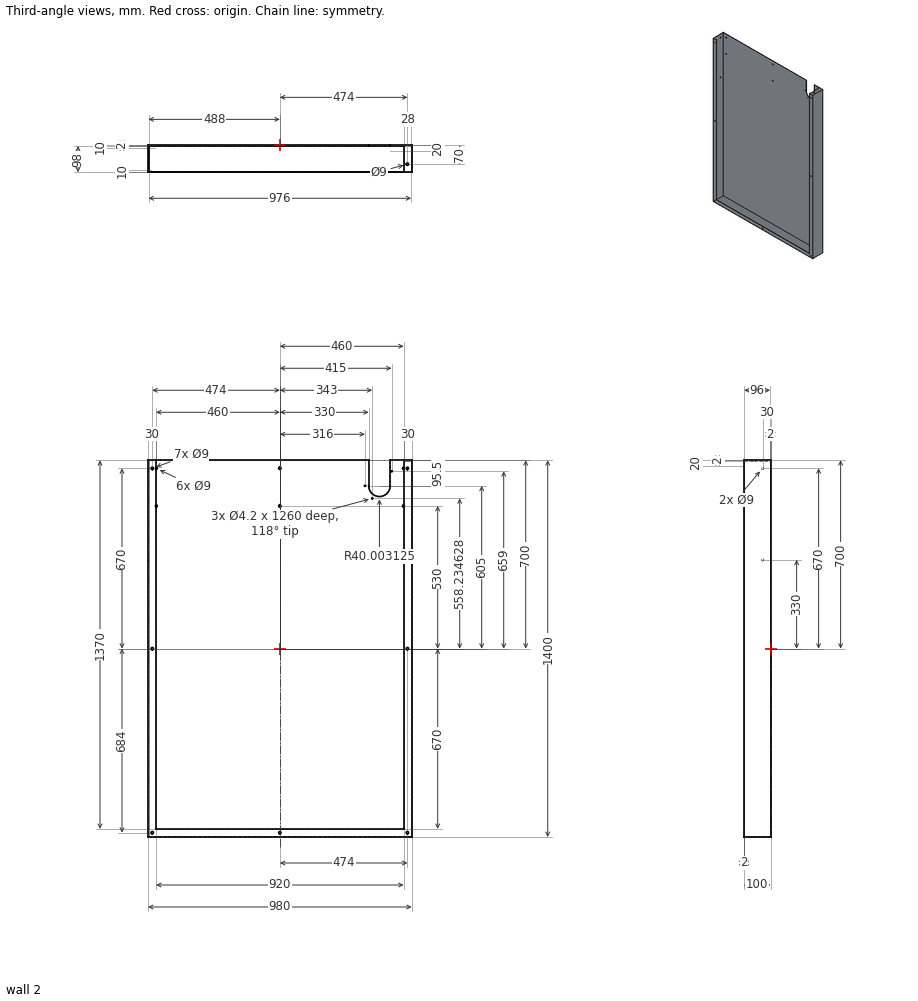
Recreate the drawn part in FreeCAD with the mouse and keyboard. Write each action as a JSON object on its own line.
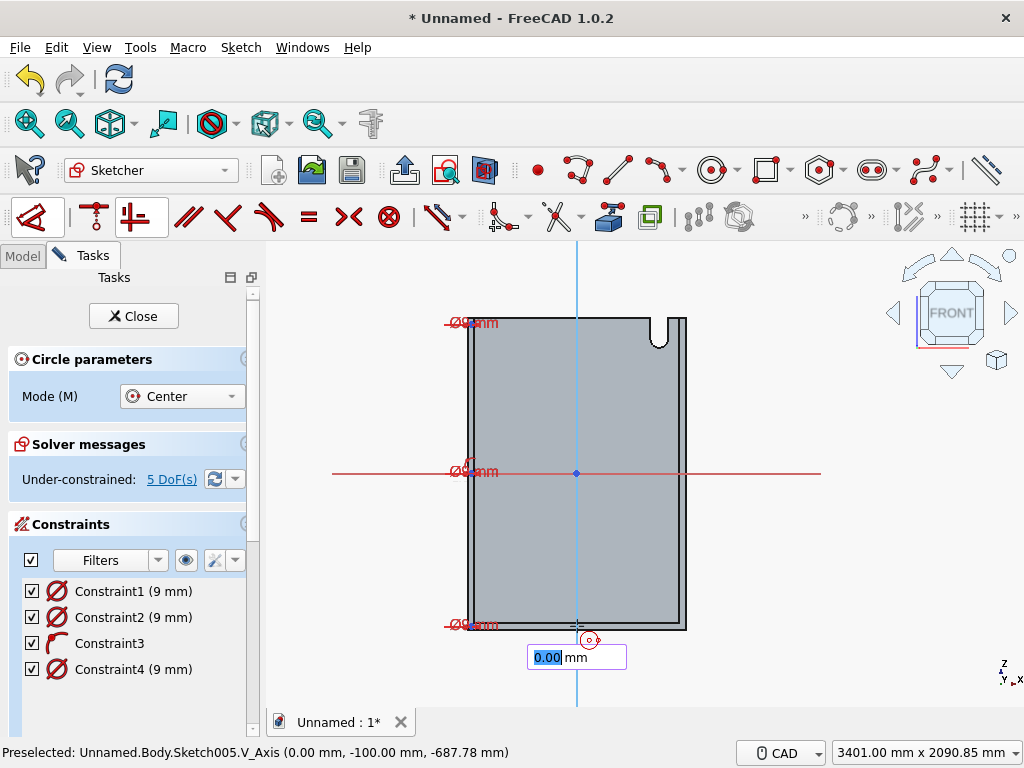
{"action": "scroll", "coordinate": [578, 626], "scroll_direction": "up", "scroll_amount": 15}
{"action": "mouse_move", "coordinate": [565, 606]}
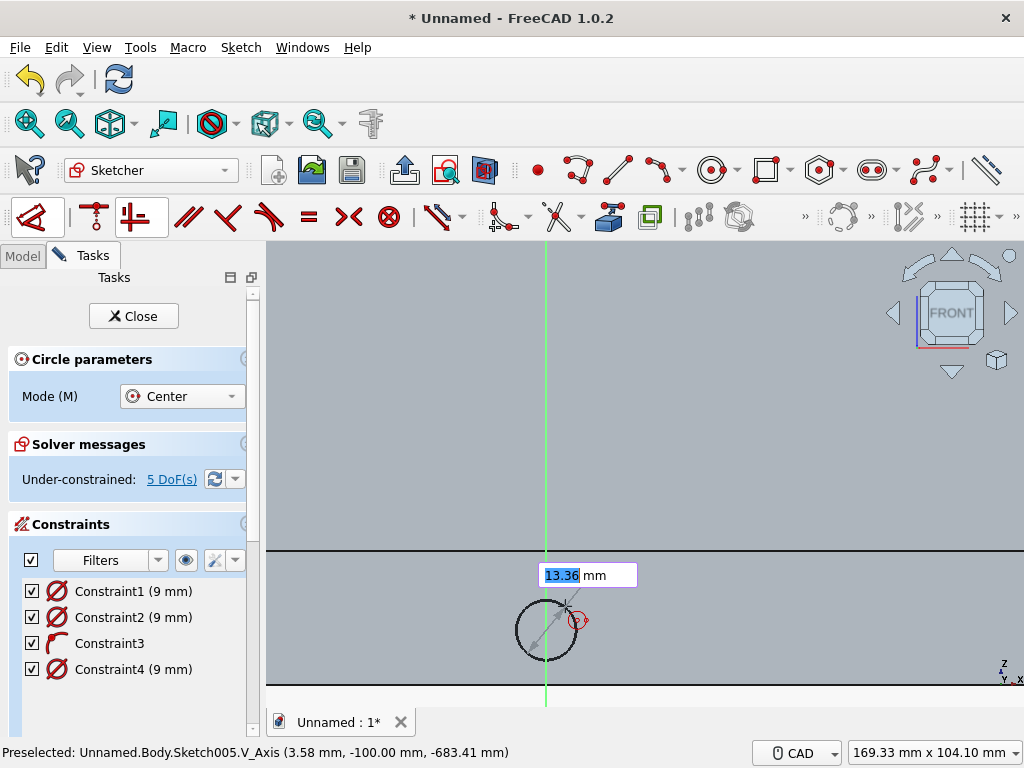
{"action": "type", "text": "9"}
{"action": "key", "text": "Return"}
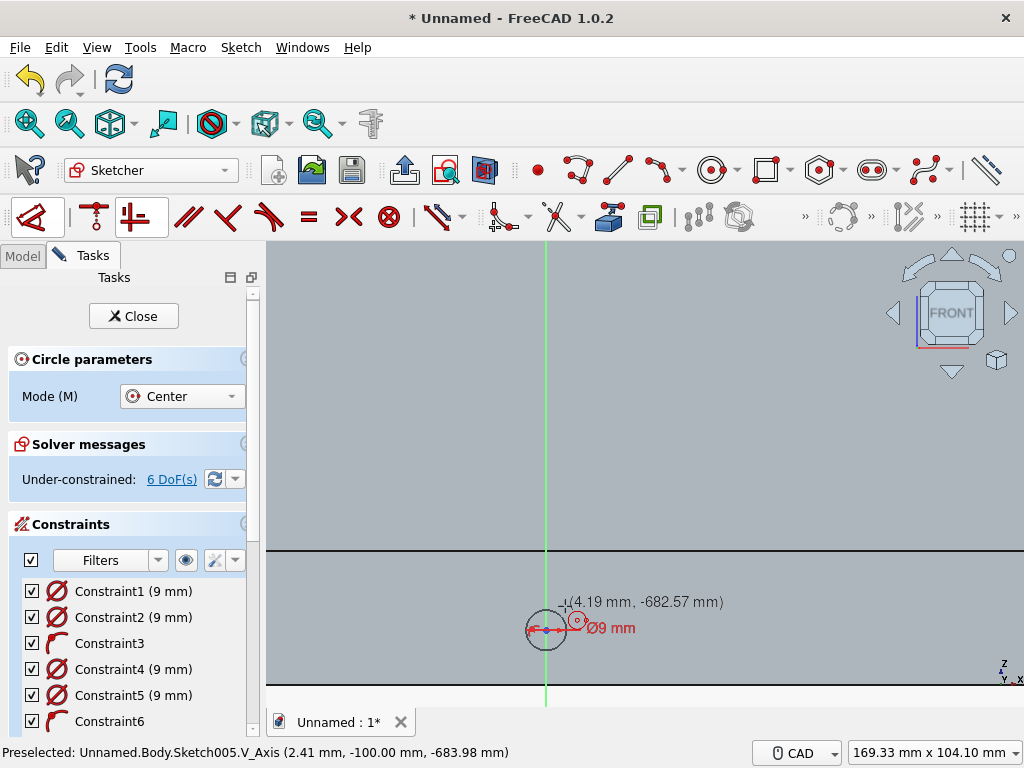
{"action": "scroll", "coordinate": [578, 625], "scroll_direction": "down", "scroll_amount": 15}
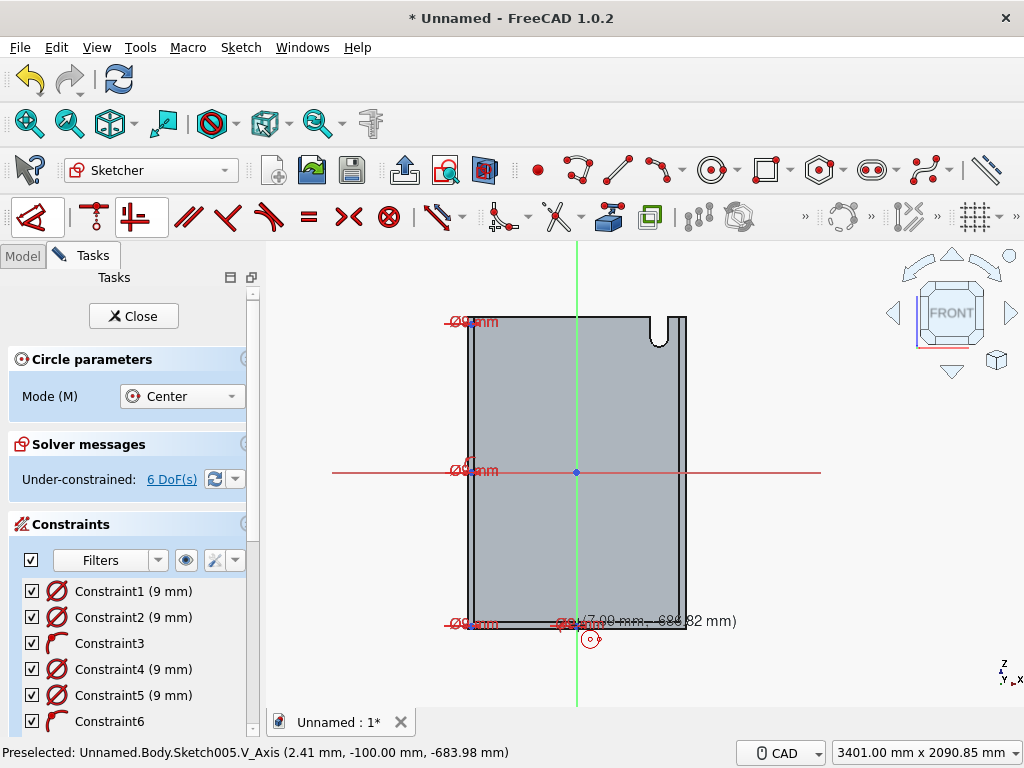
{"action": "scroll", "coordinate": [682, 625], "scroll_direction": "up", "scroll_amount": 16}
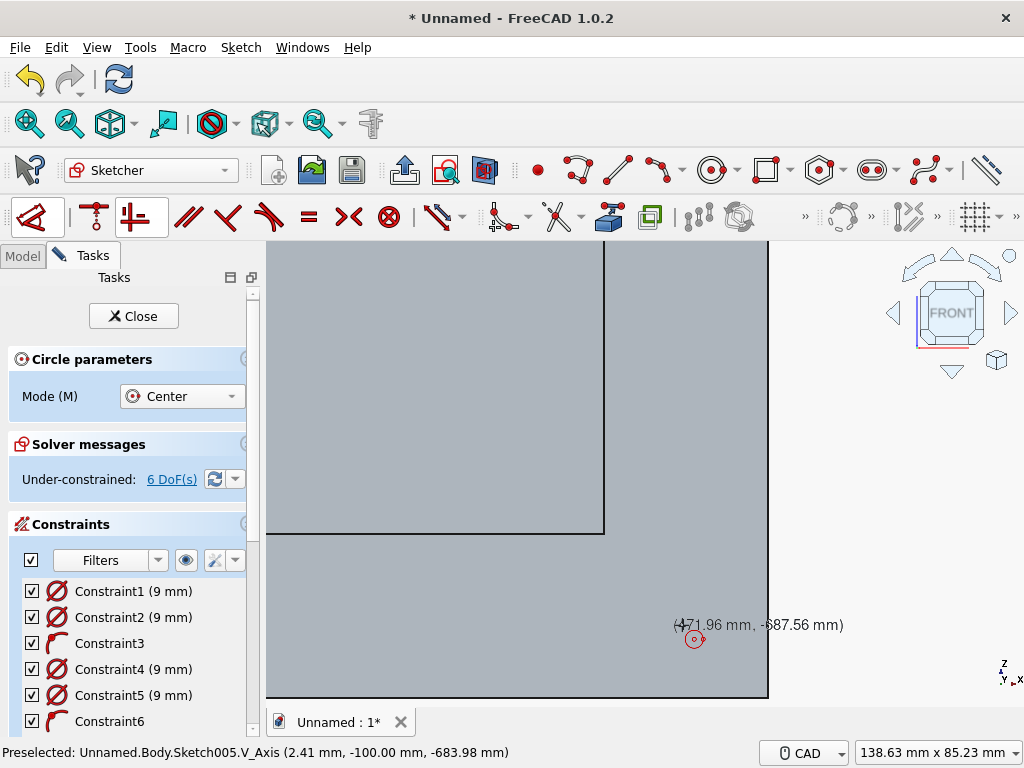
{"action": "scroll", "coordinate": [682, 625], "scroll_direction": "down", "scroll_amount": 16}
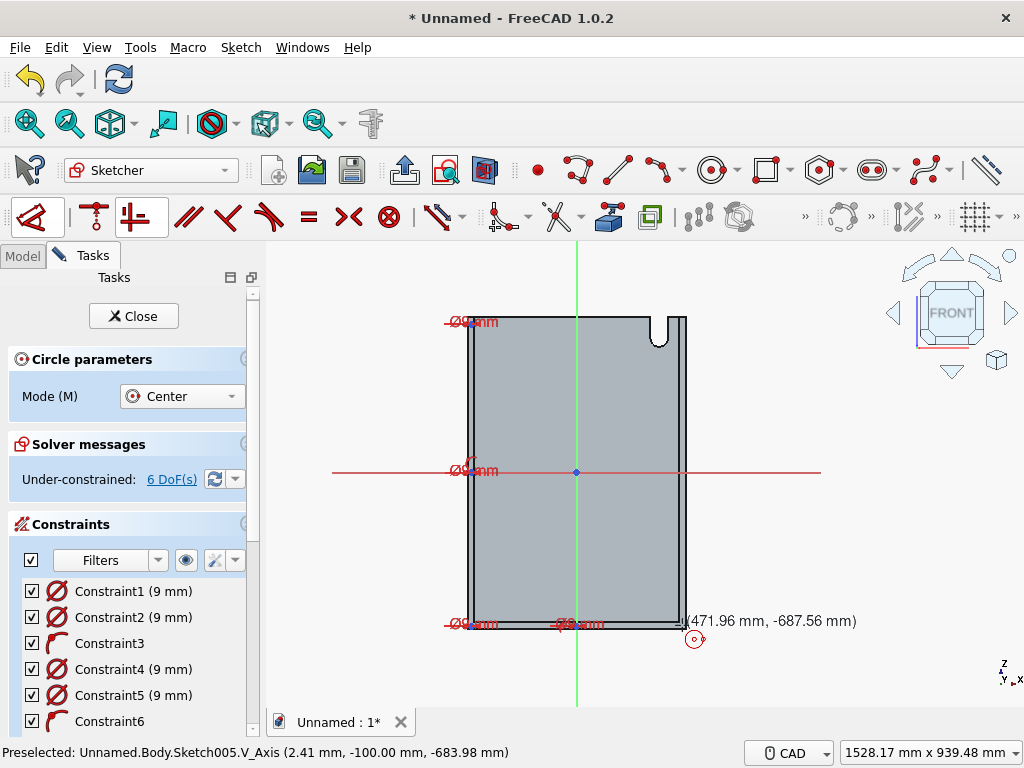
{"action": "left_click", "coordinate": [682, 625]}
{"action": "mouse_move", "coordinate": [683, 624]}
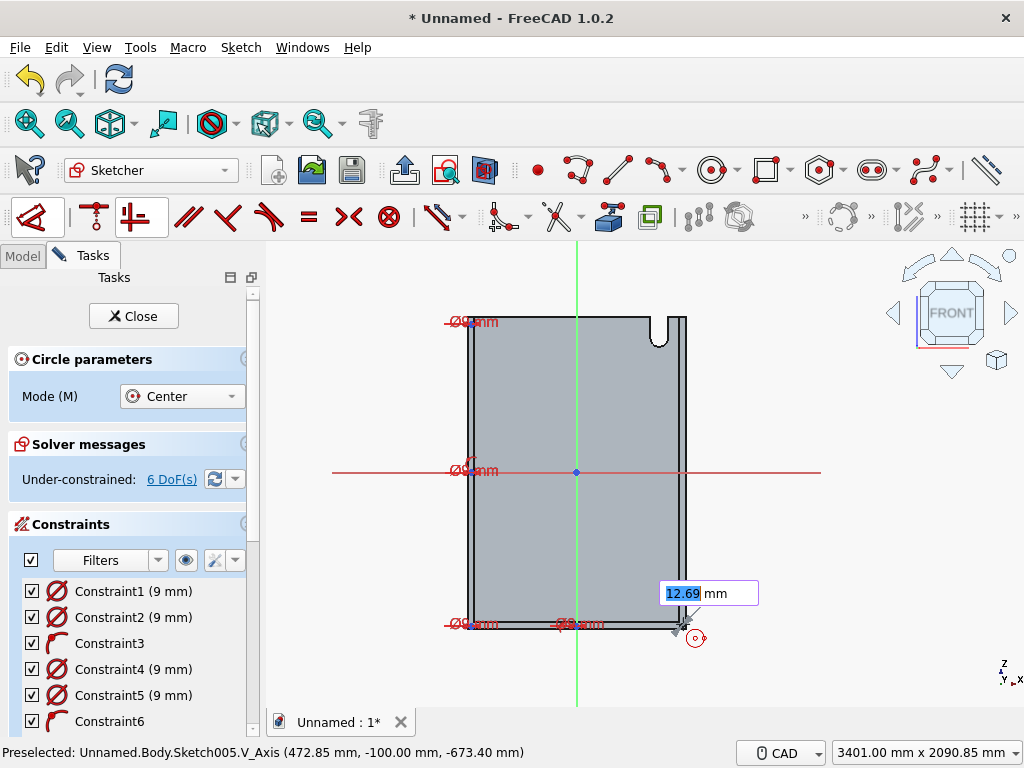
{"action": "type", "text": "9"}
{"action": "key", "text": "Return"}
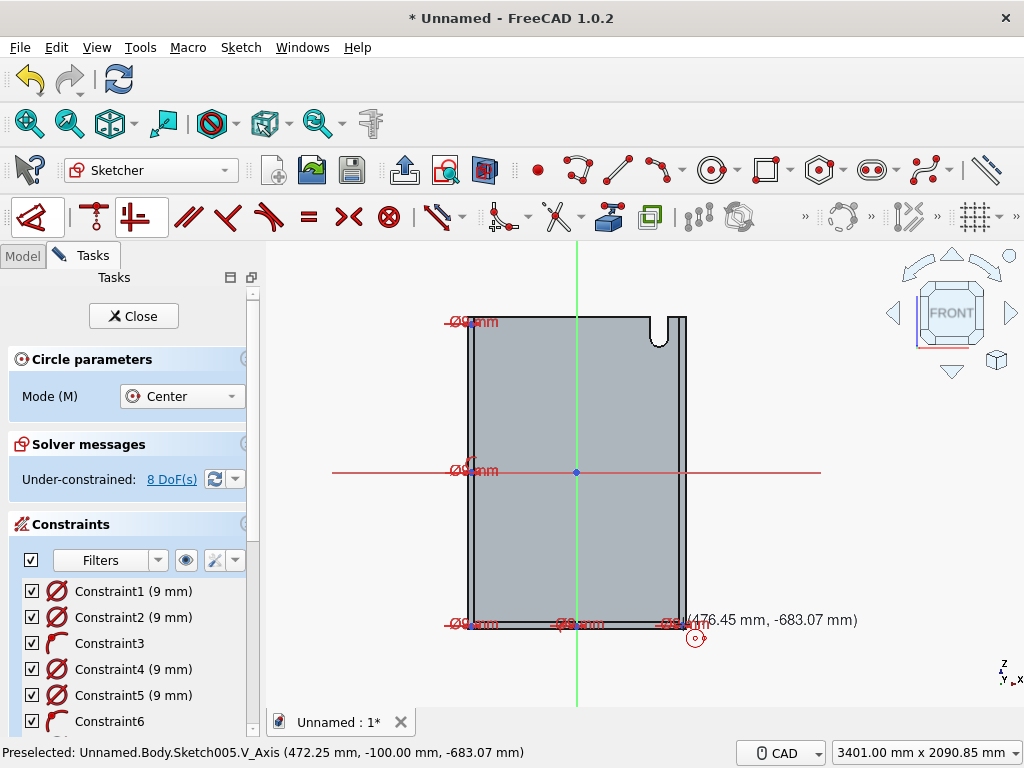
{"action": "scroll", "coordinate": [682, 473], "scroll_direction": "up", "scroll_amount": 16}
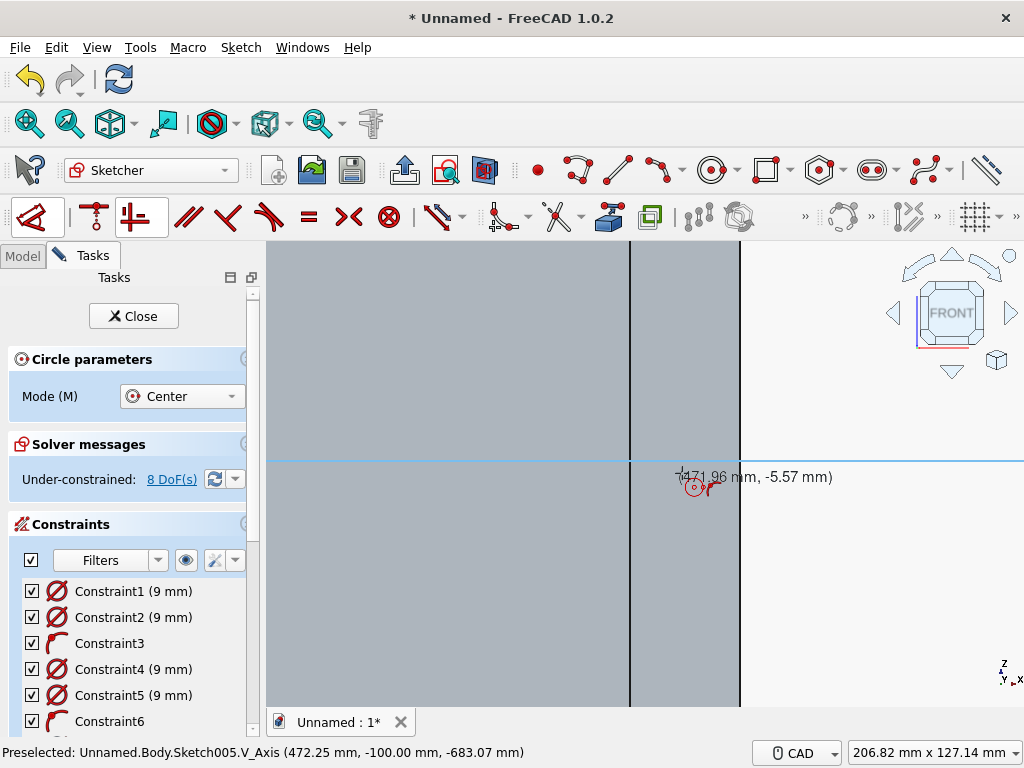
{"action": "scroll", "coordinate": [682, 473], "scroll_direction": "down", "scroll_amount": 16}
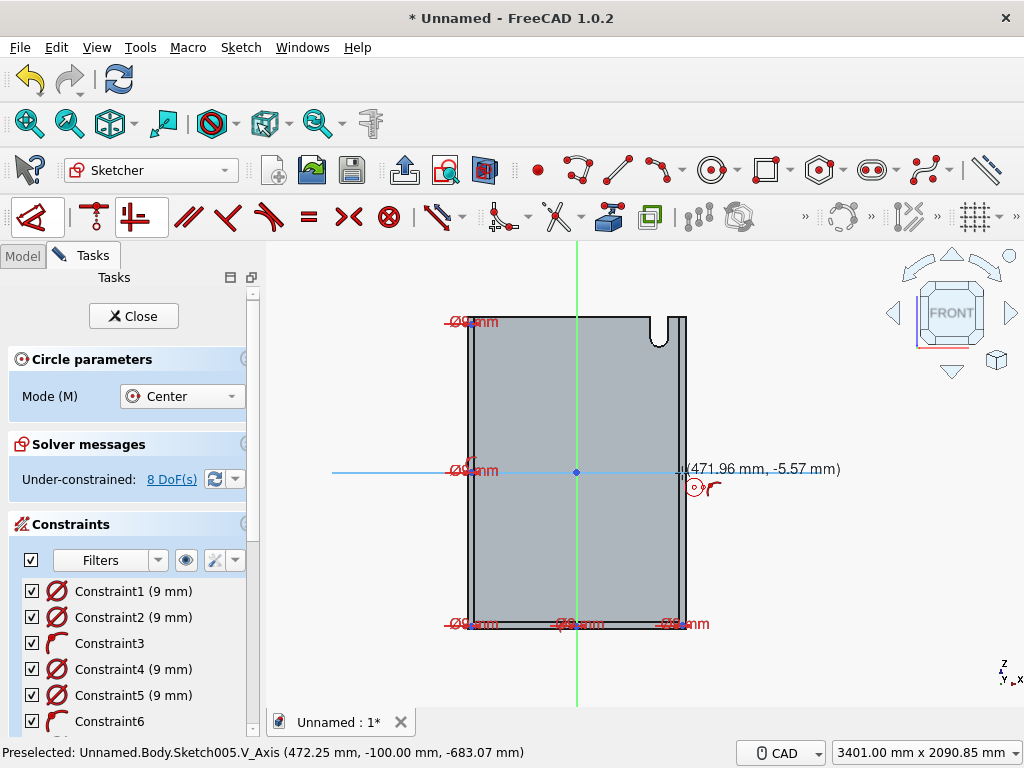
{"action": "left_click", "coordinate": [682, 473]}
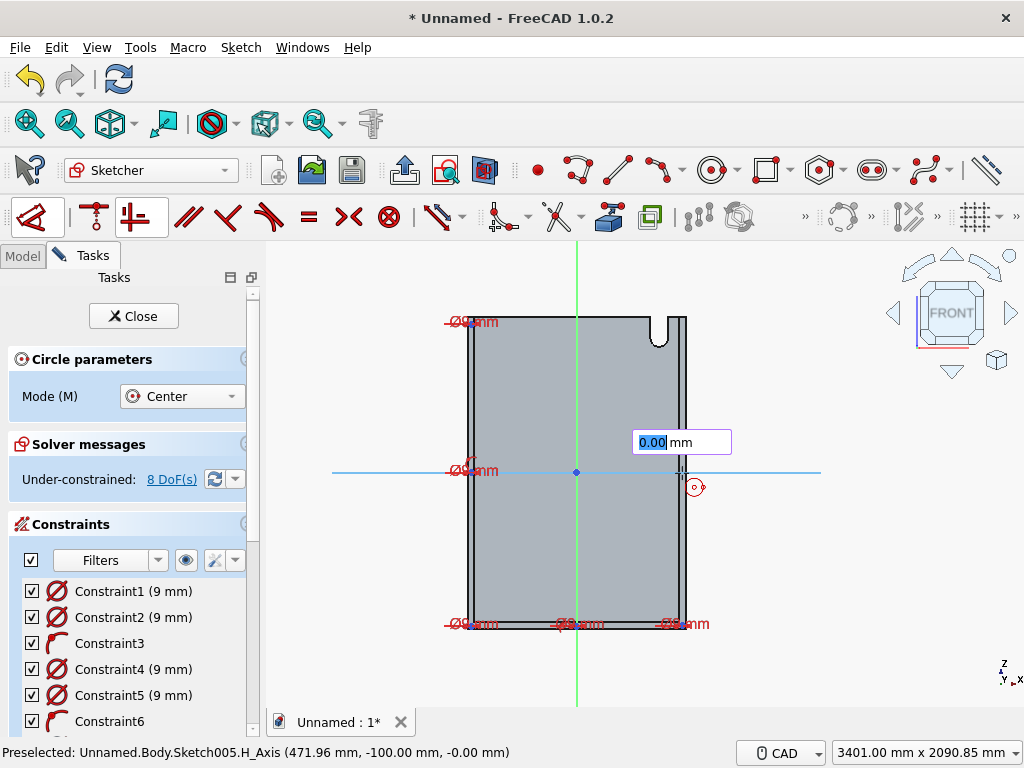
{"action": "scroll", "coordinate": [682, 474], "scroll_direction": "up", "scroll_amount": 15}
{"action": "mouse_move", "coordinate": [674, 458]}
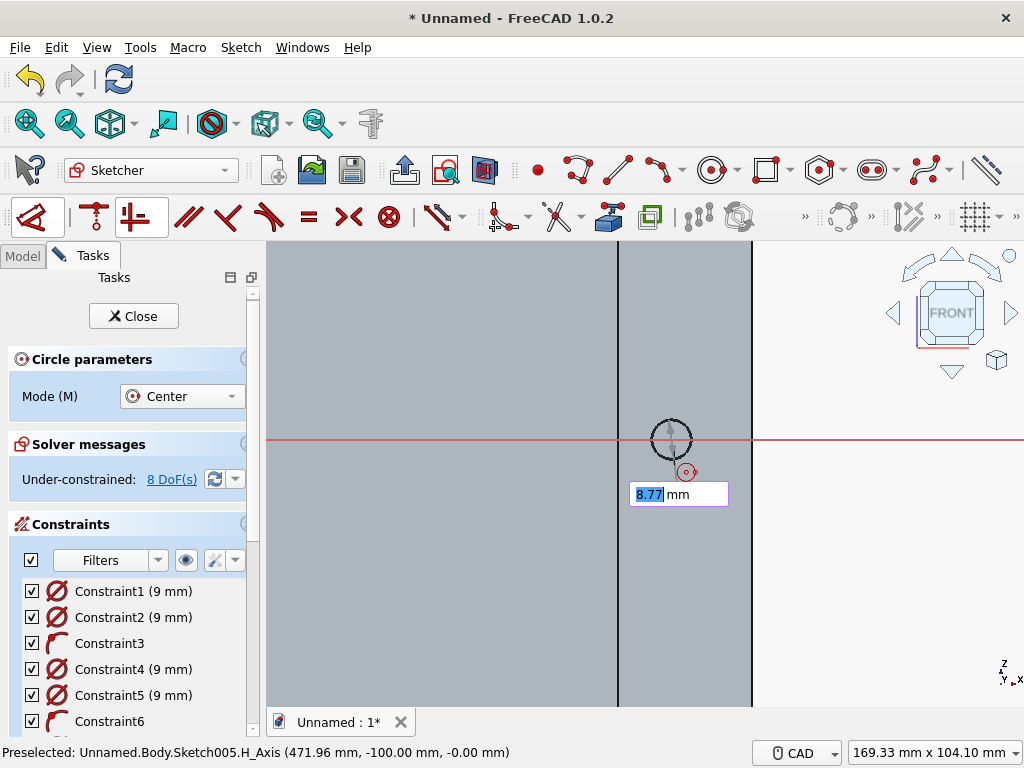
{"action": "type", "text": "9"}
{"action": "key", "text": "Return"}